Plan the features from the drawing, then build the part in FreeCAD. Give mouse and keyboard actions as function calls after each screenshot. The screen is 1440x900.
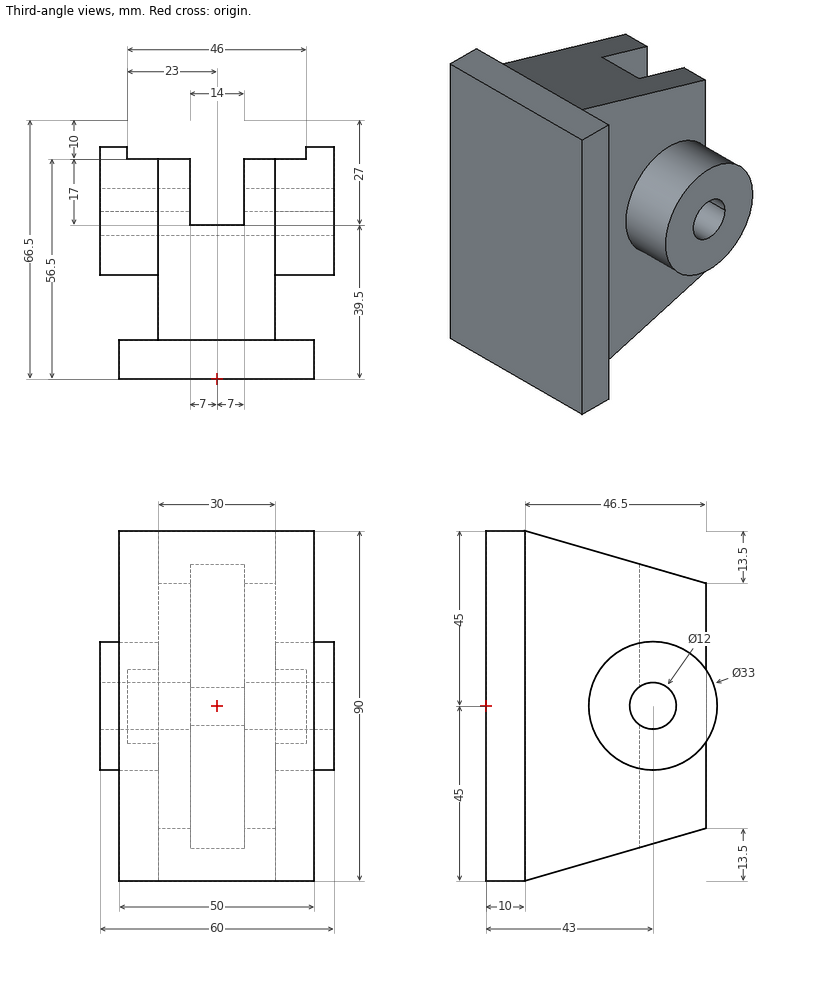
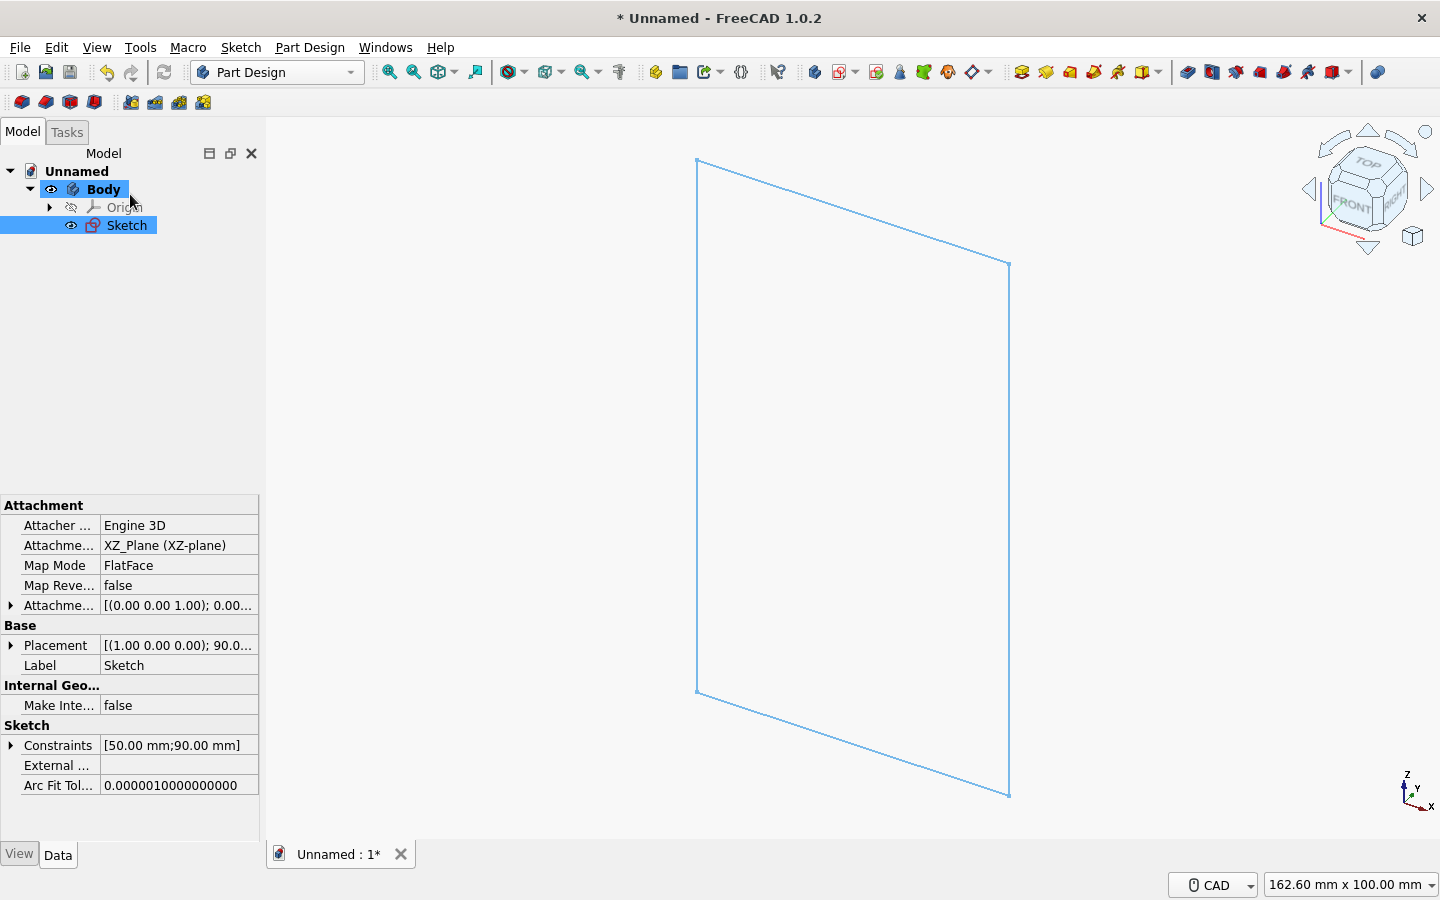
click(1022, 72)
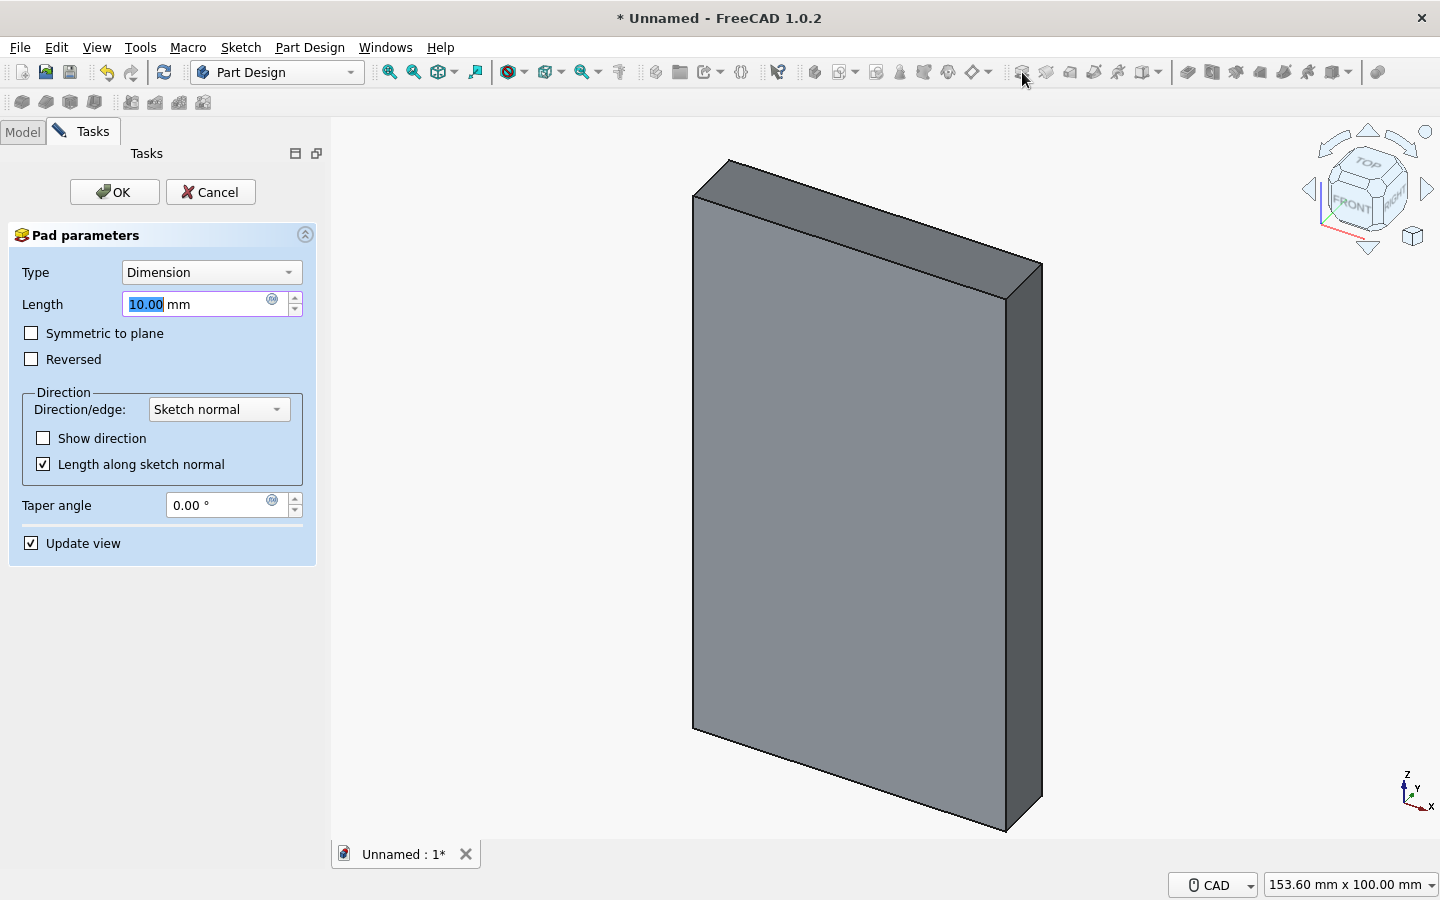
text(10)
key(Tab)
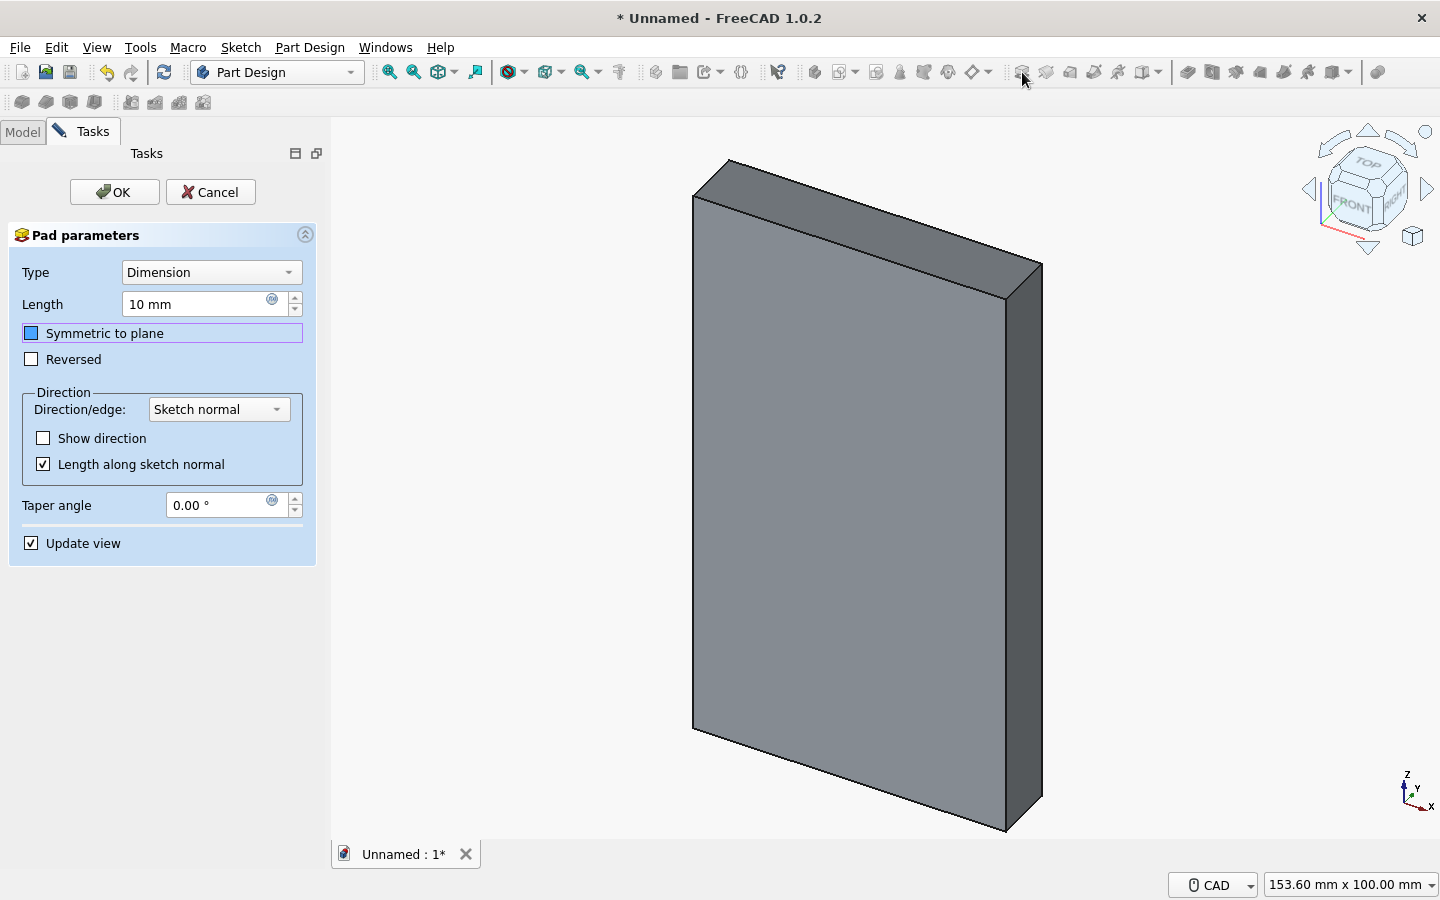
click(30, 359)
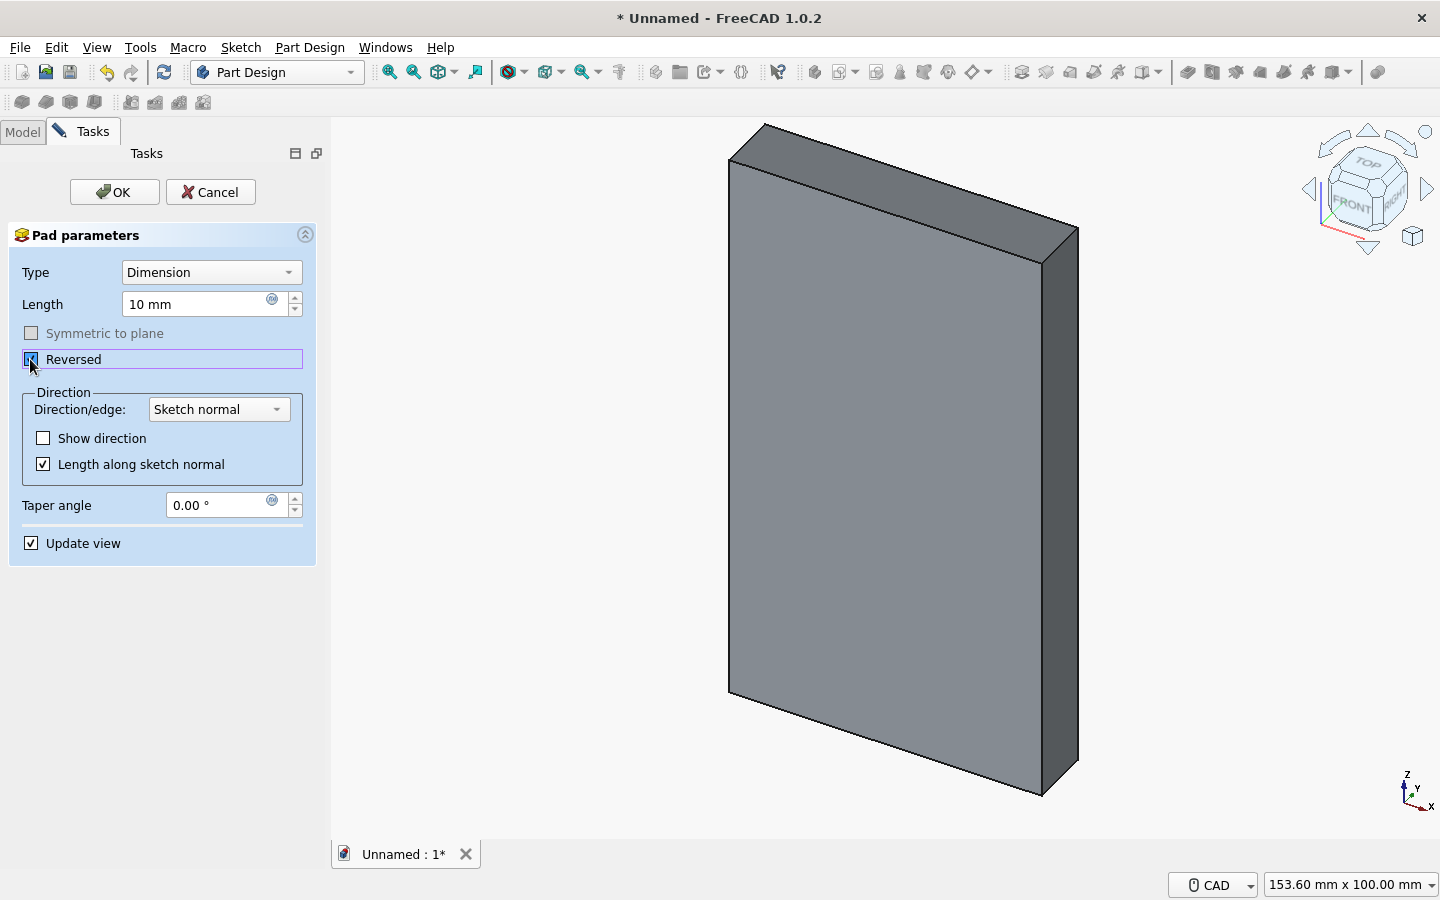
click(115, 192)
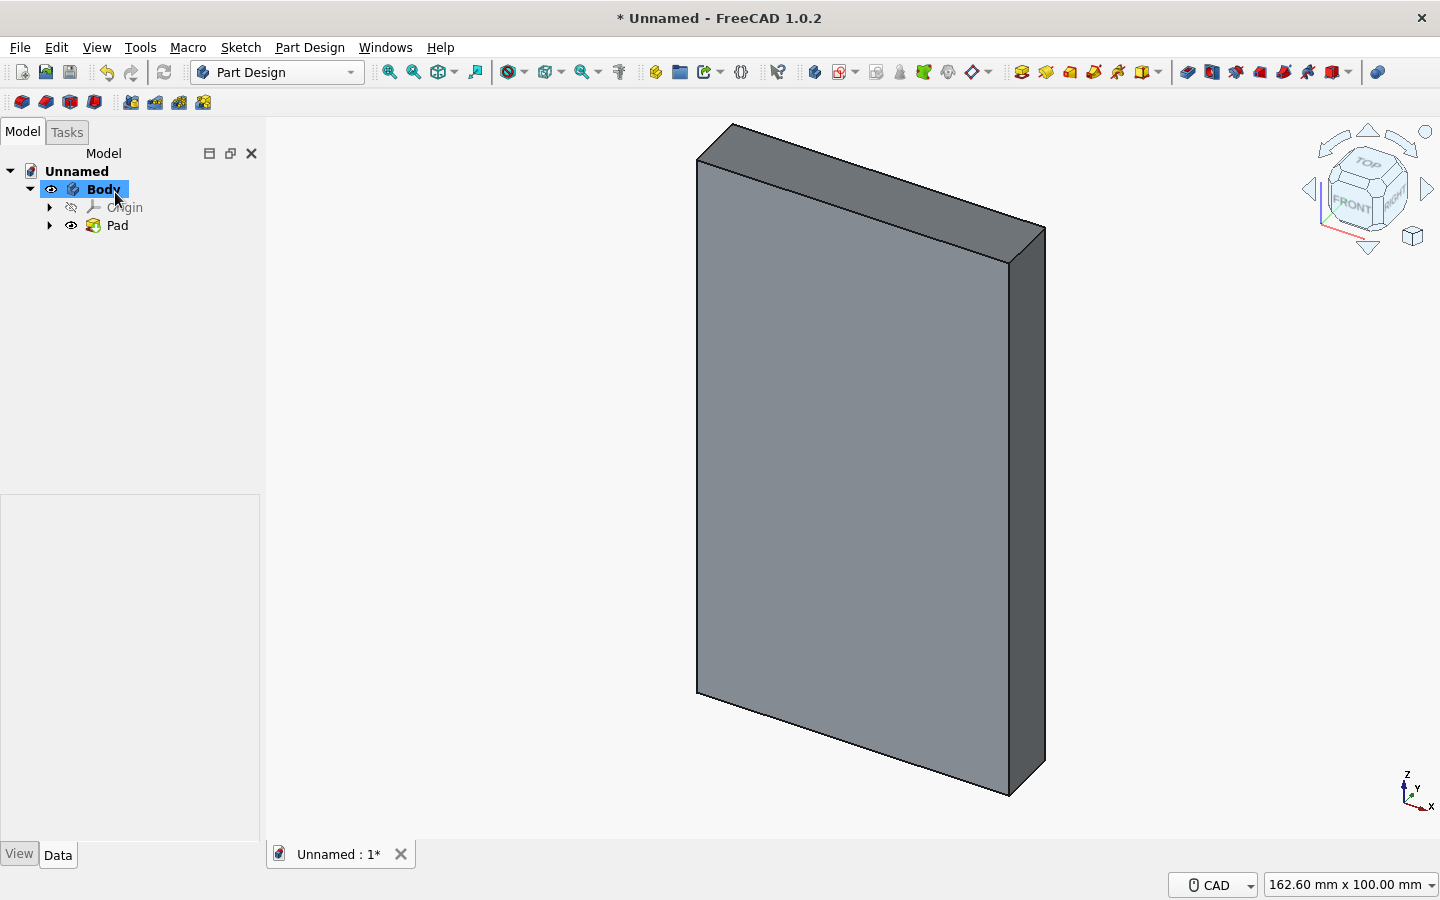
key(4)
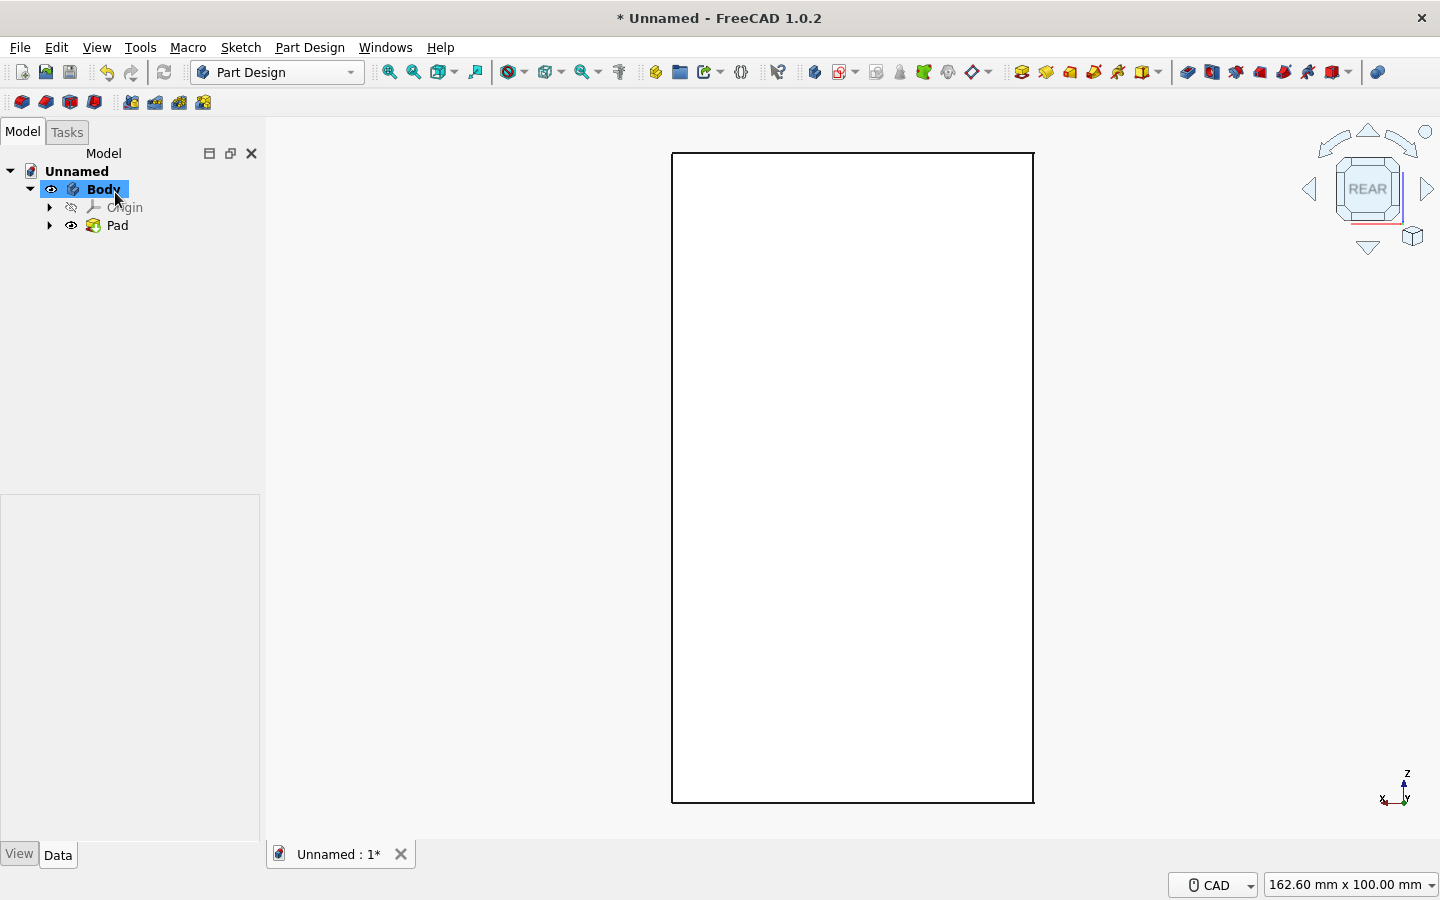
click(853, 384)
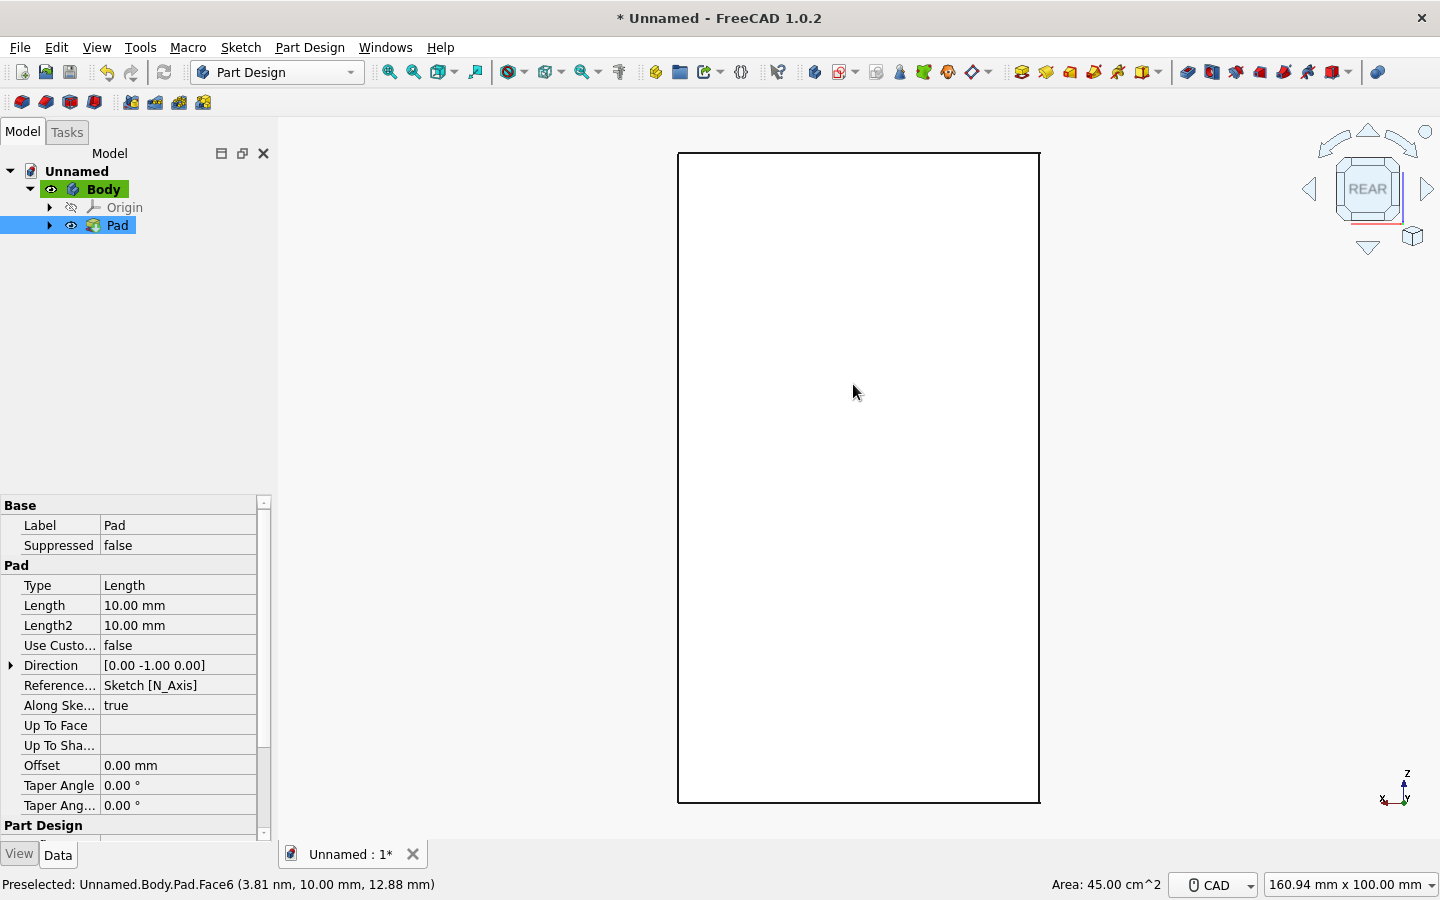
click(840, 72)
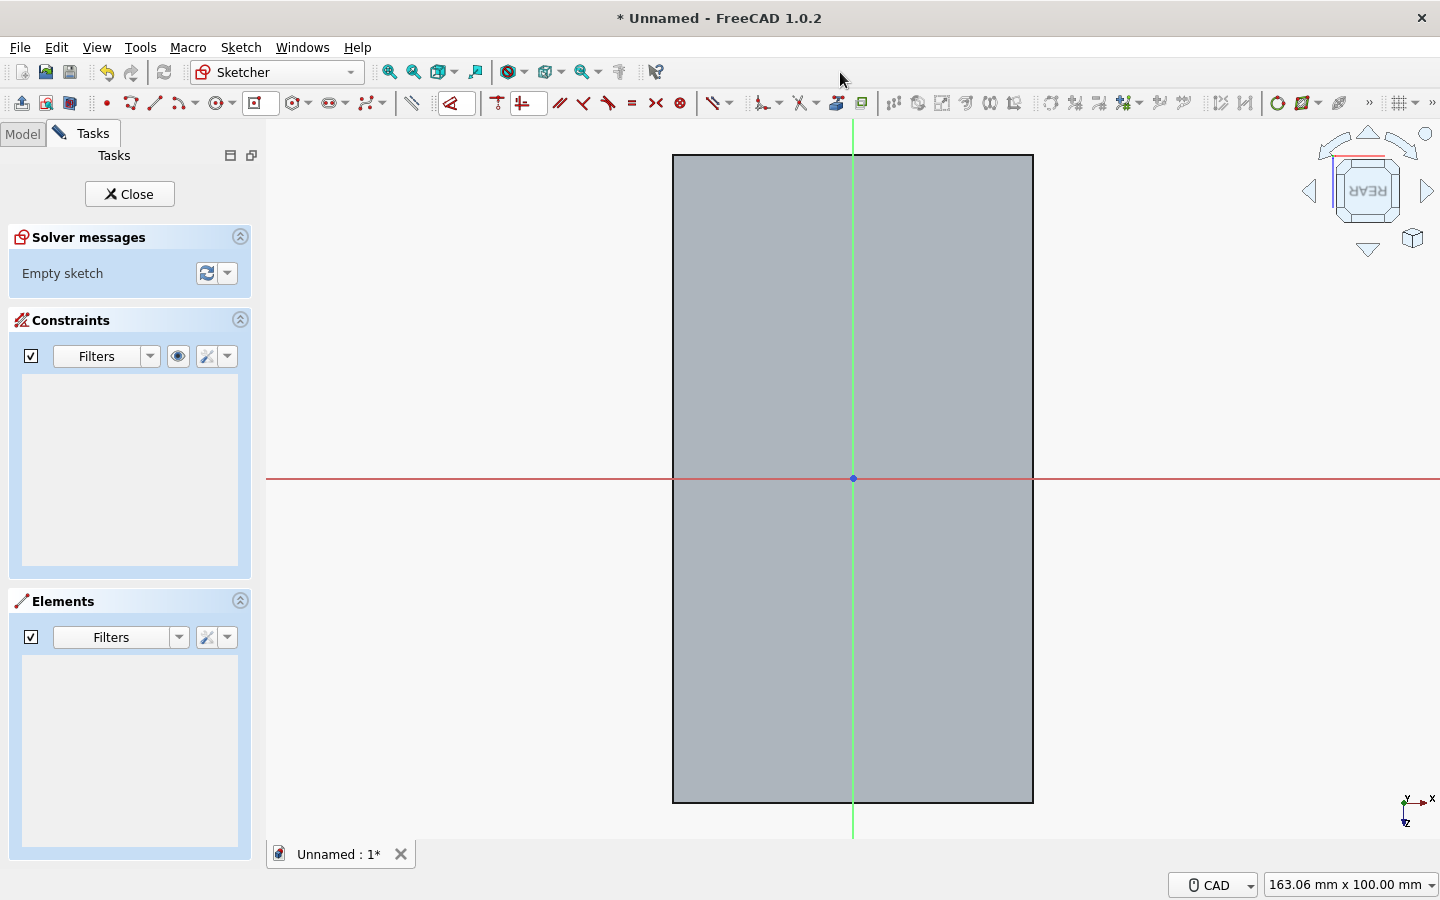
scroll(645, 479, down, 2)